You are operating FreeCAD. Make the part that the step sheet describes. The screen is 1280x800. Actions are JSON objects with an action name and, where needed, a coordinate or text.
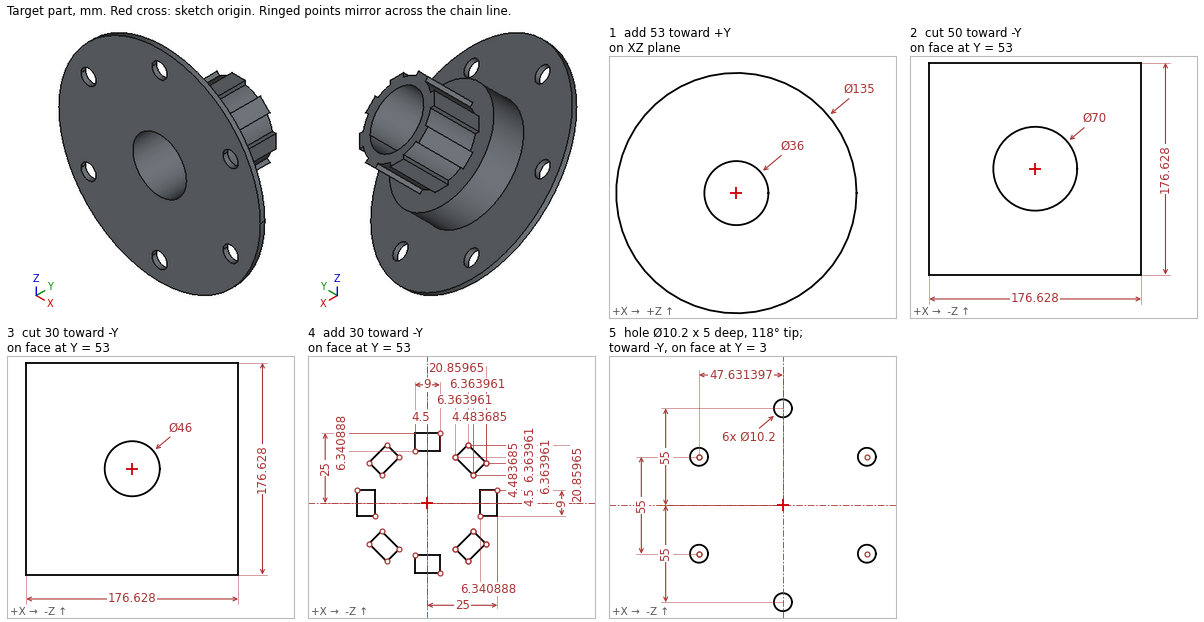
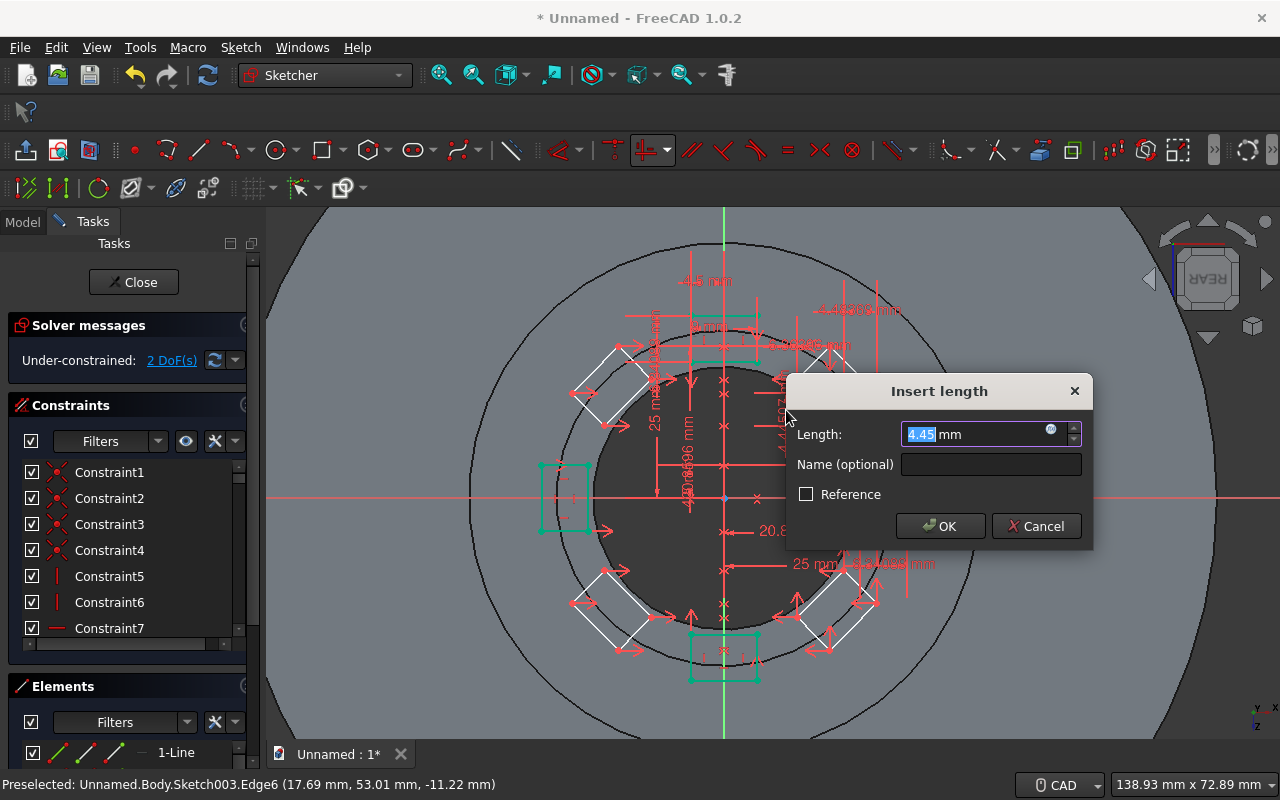
{"action": "type", "text": "4.483685"}
{"action": "key", "text": "Return"}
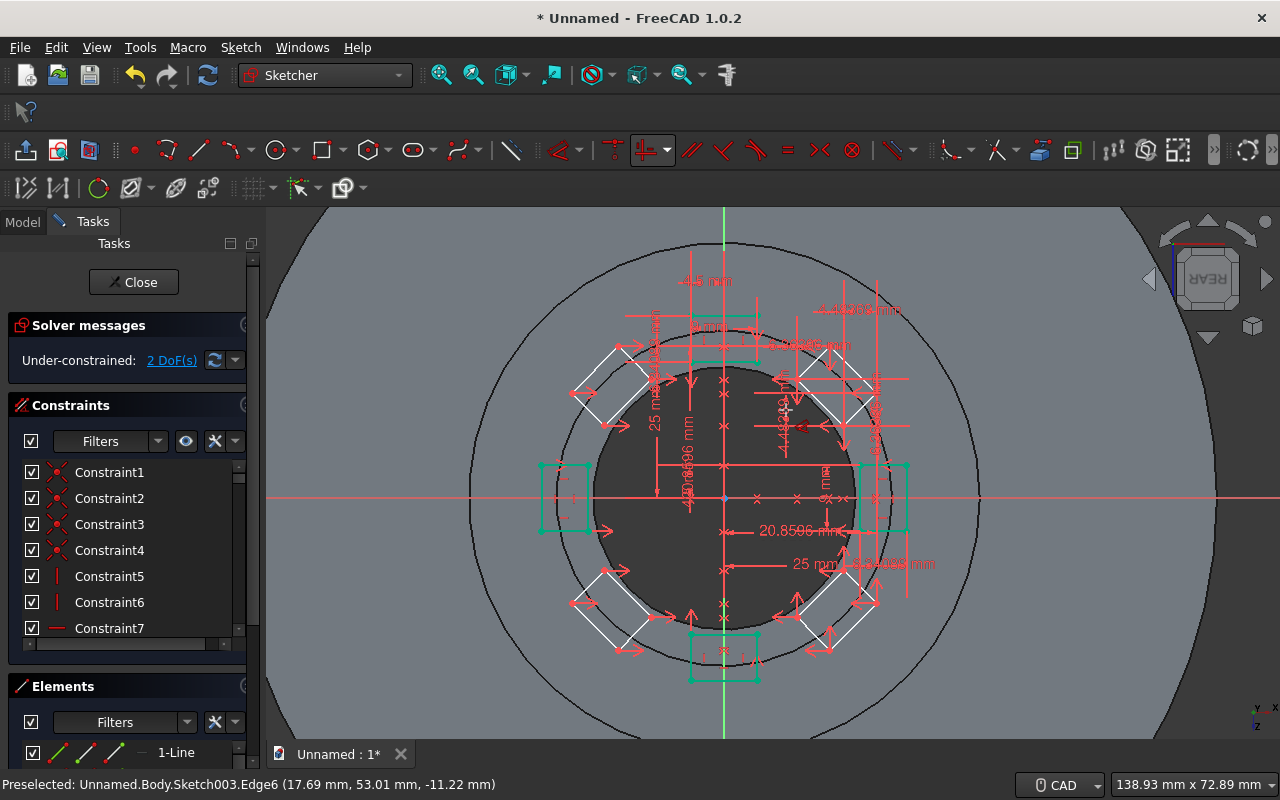
{"action": "left_click", "coordinate": [863, 379]}
{"action": "left_click", "coordinate": [853, 288]}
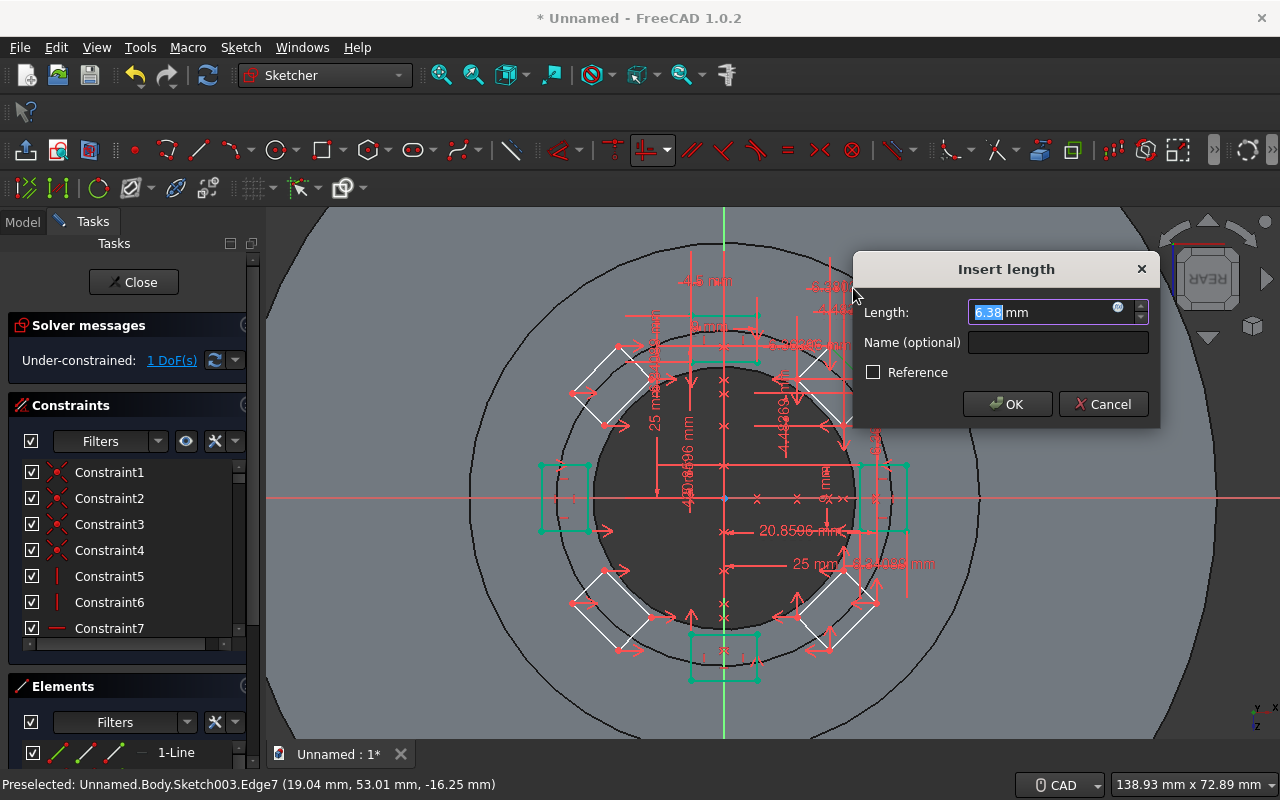
{"action": "type", "text": "6.363961"}
{"action": "key", "text": "Return"}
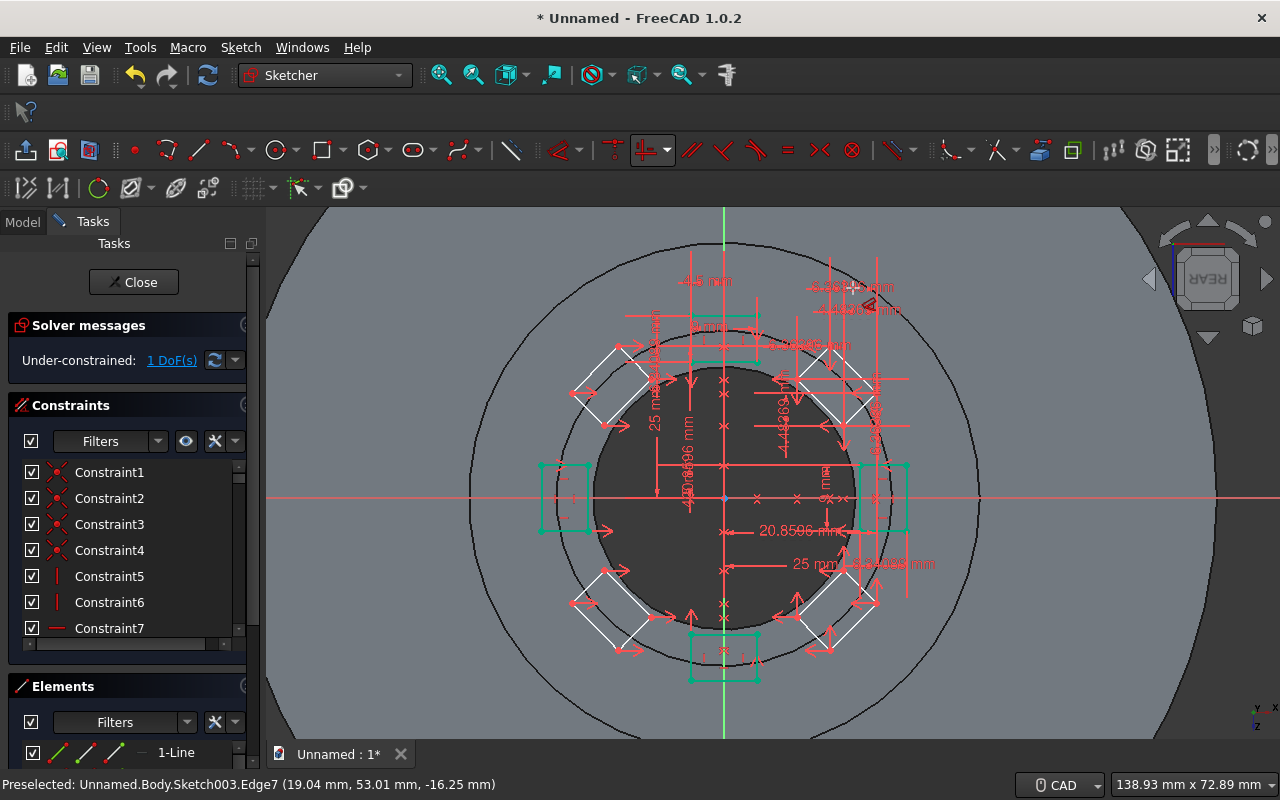
{"action": "left_click", "coordinate": [863, 379]}
{"action": "left_click", "coordinate": [911, 370]}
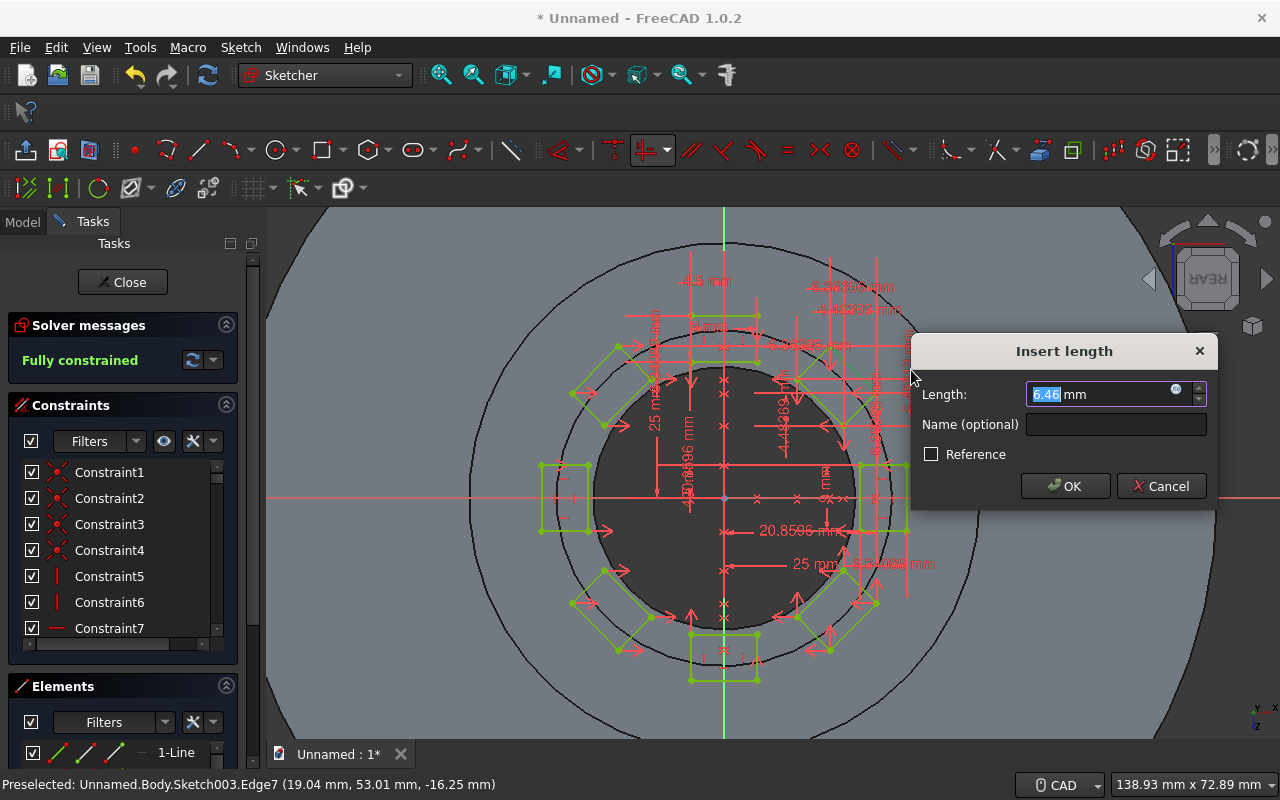
{"action": "type", "text": "6.363961"}
{"action": "key", "text": "Return"}
{"action": "key", "text": "Escape"}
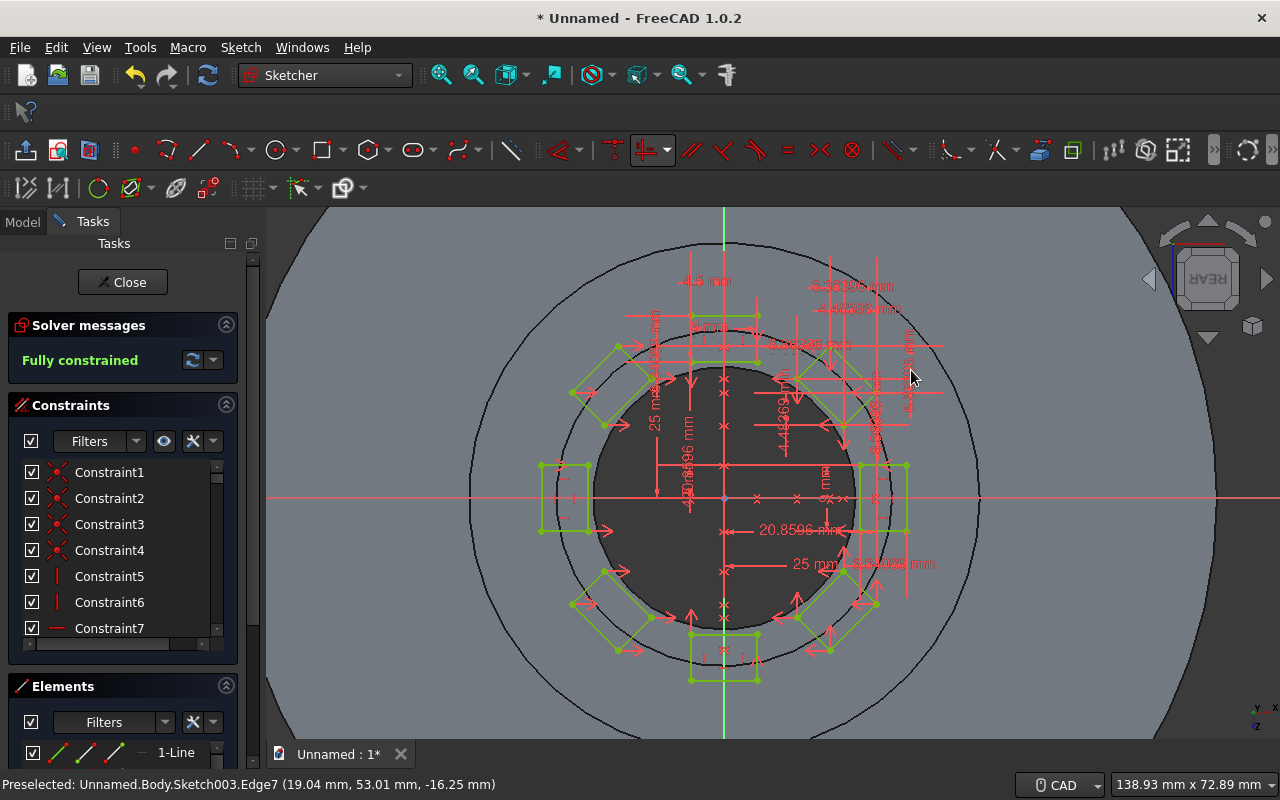
{"action": "left_click", "coordinate": [123, 282]}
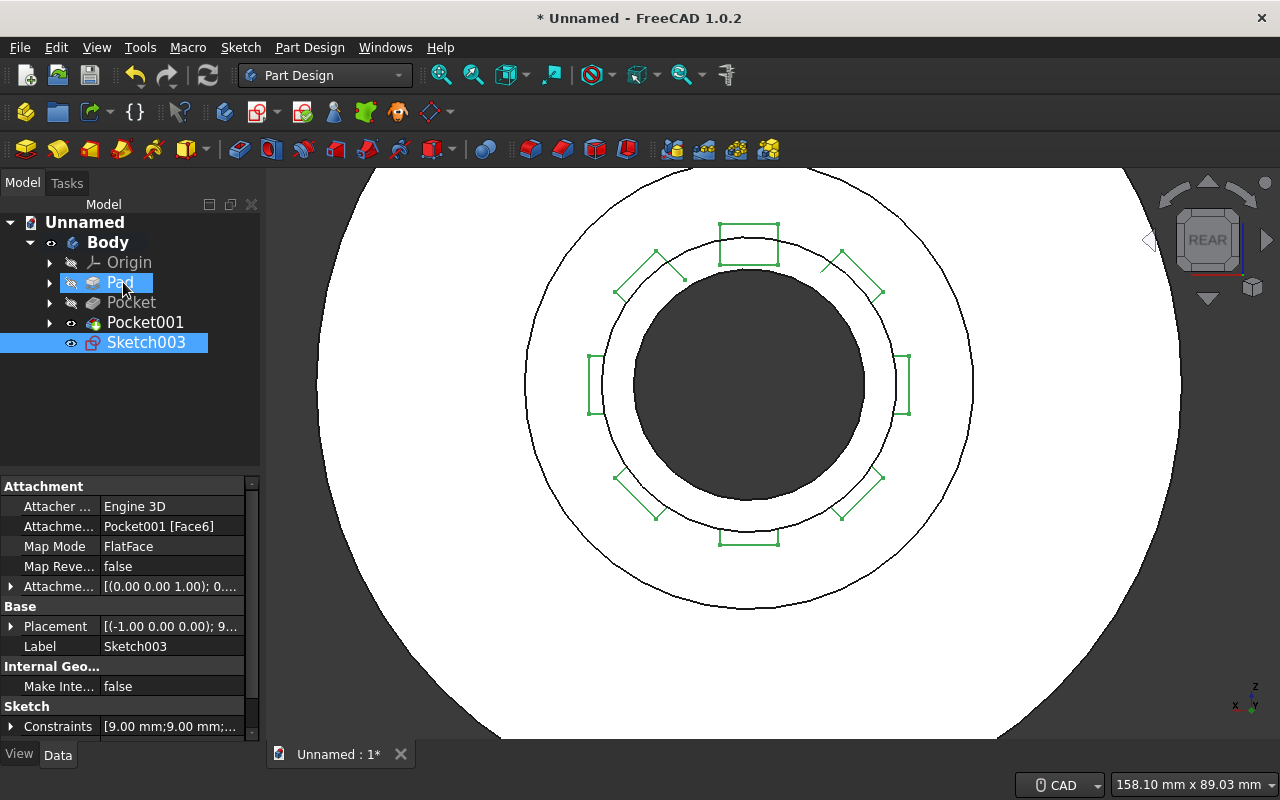
{"action": "left_click", "coordinate": [26, 150]}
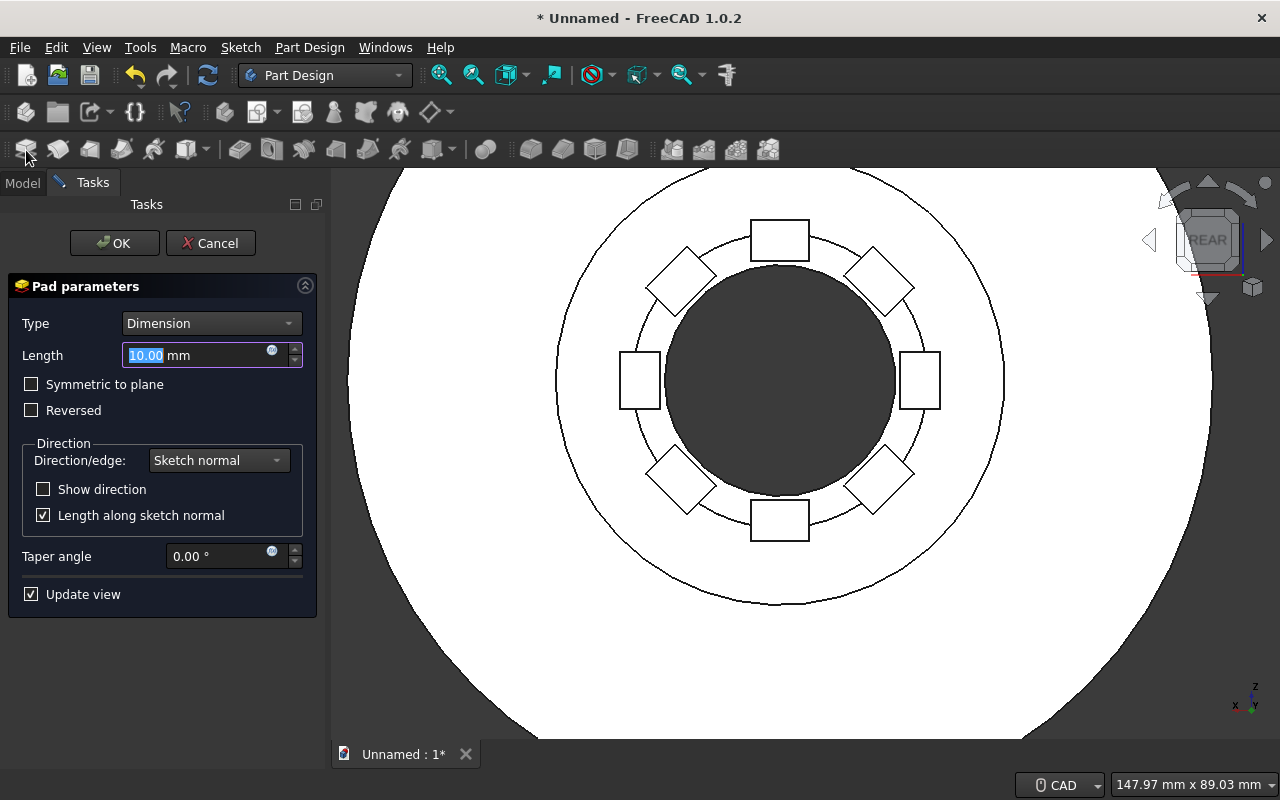
{"action": "type", "text": "30"}
{"action": "key", "text": "Tab"}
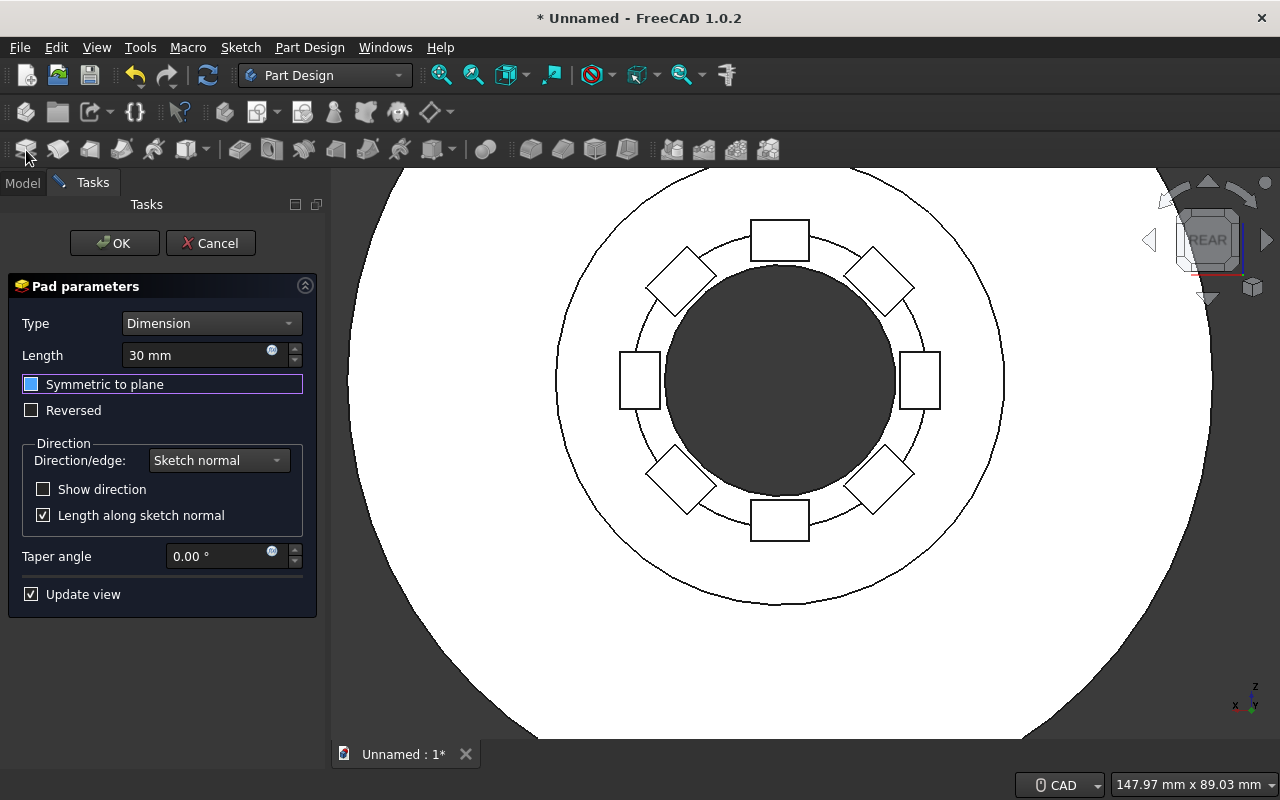
{"action": "left_click", "coordinate": [30, 410]}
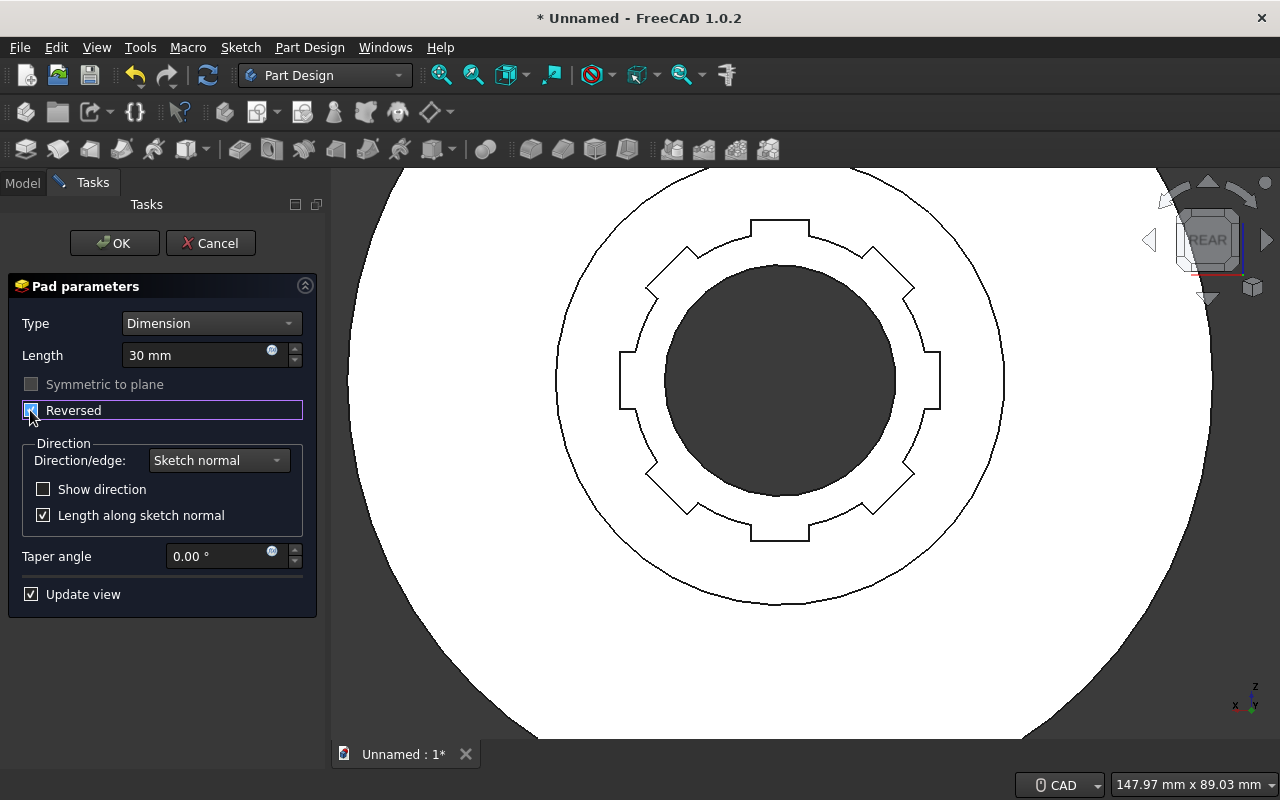
{"action": "left_click", "coordinate": [115, 243]}